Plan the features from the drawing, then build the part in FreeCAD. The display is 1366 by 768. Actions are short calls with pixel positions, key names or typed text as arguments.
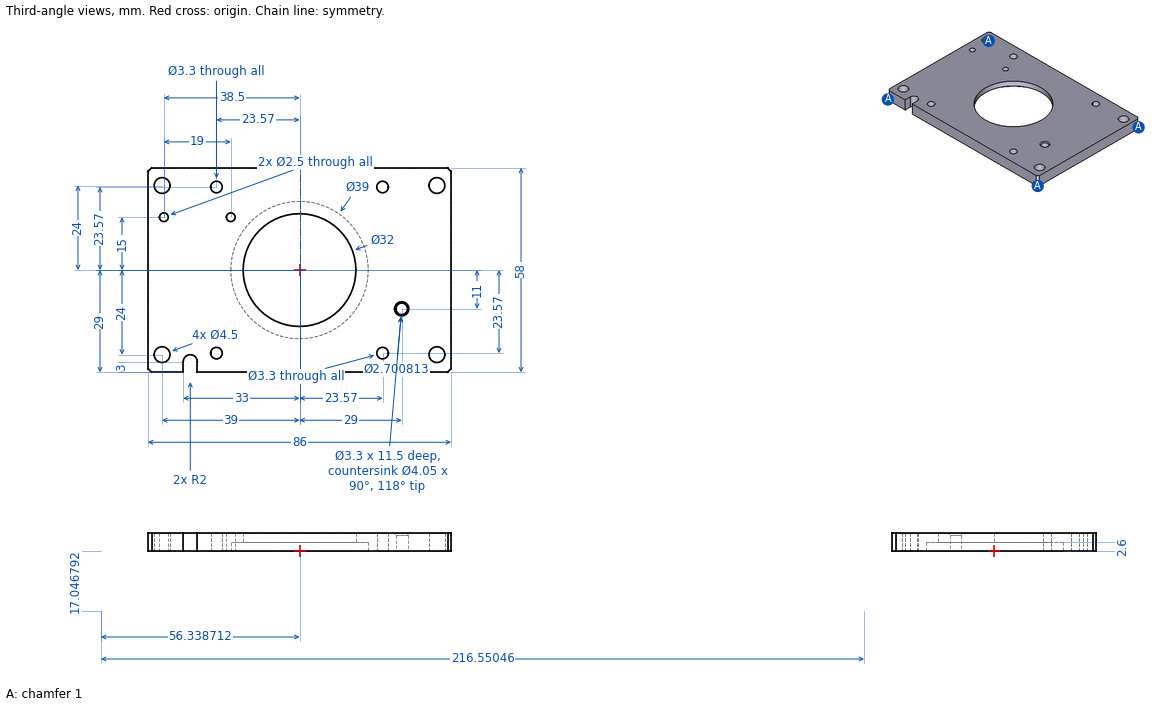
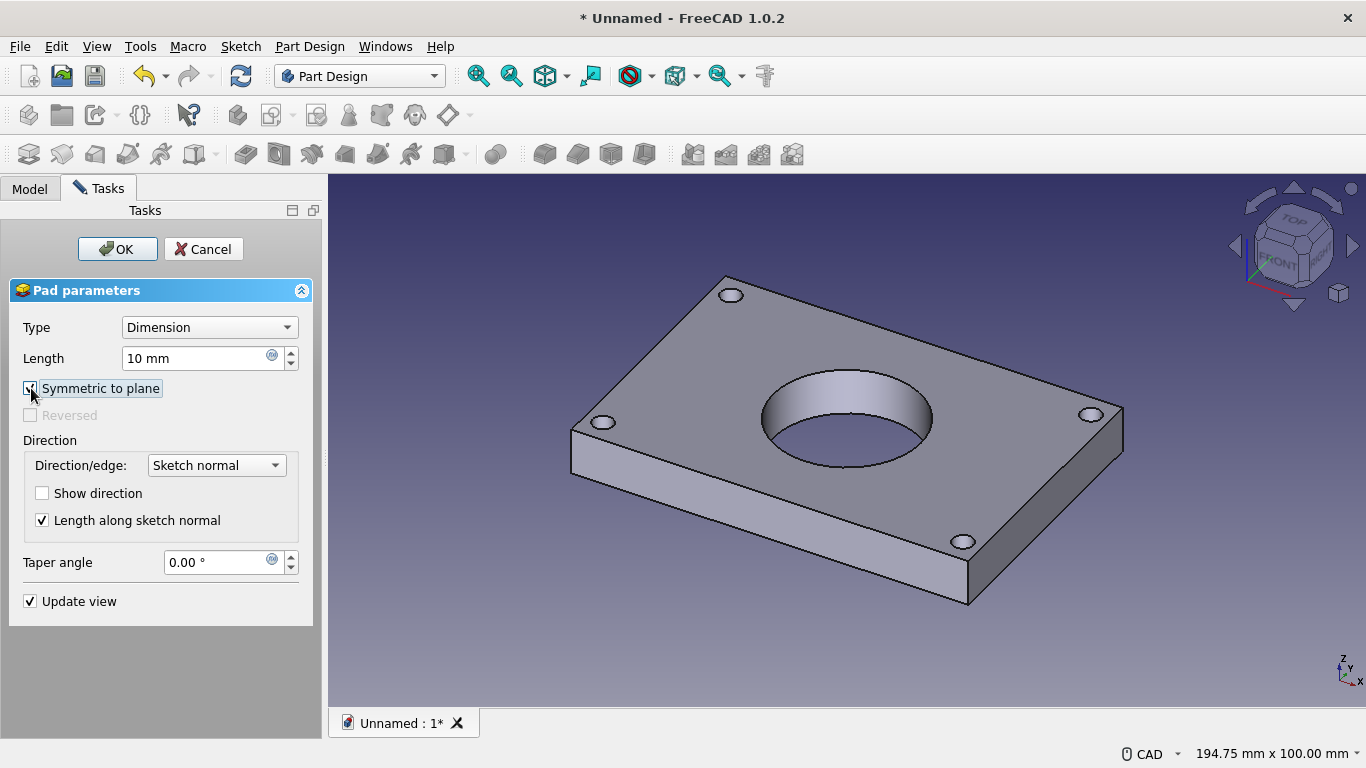
click(118, 249)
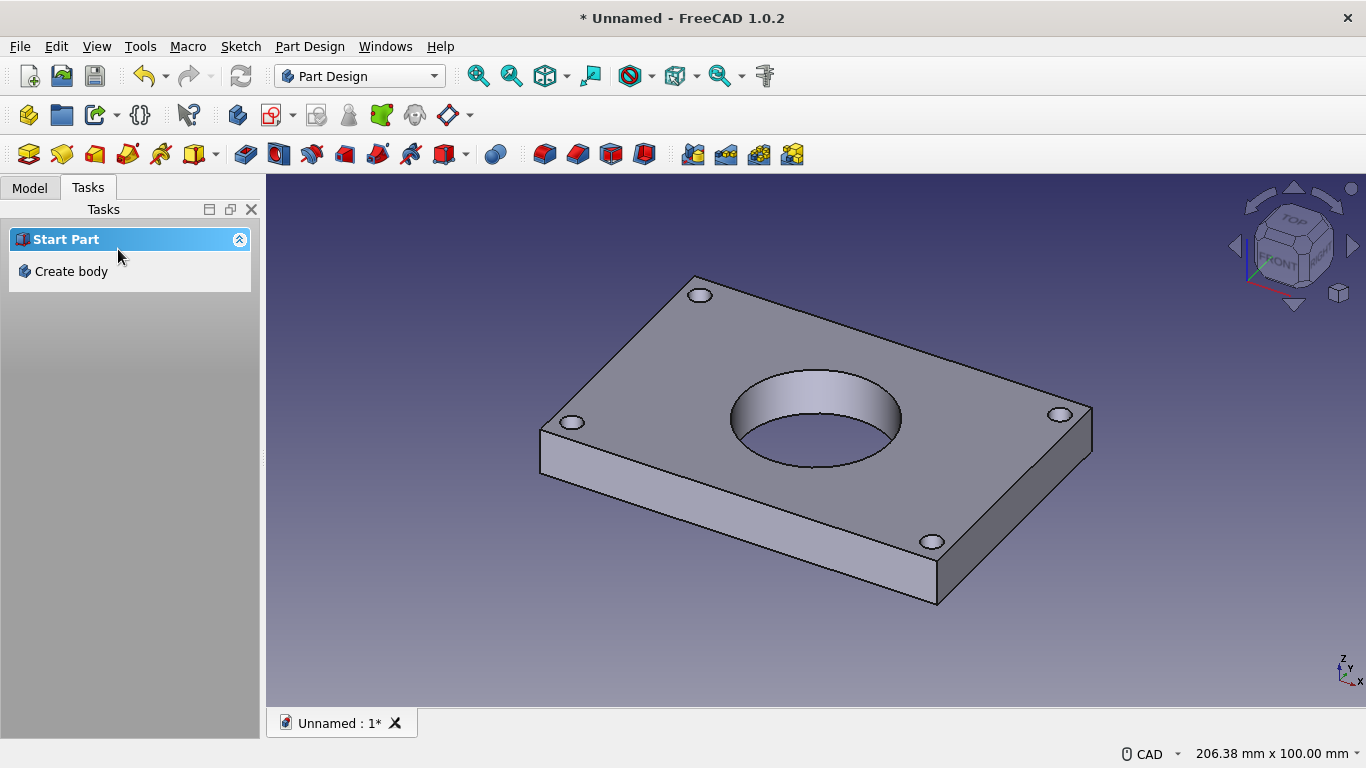
click(974, 411)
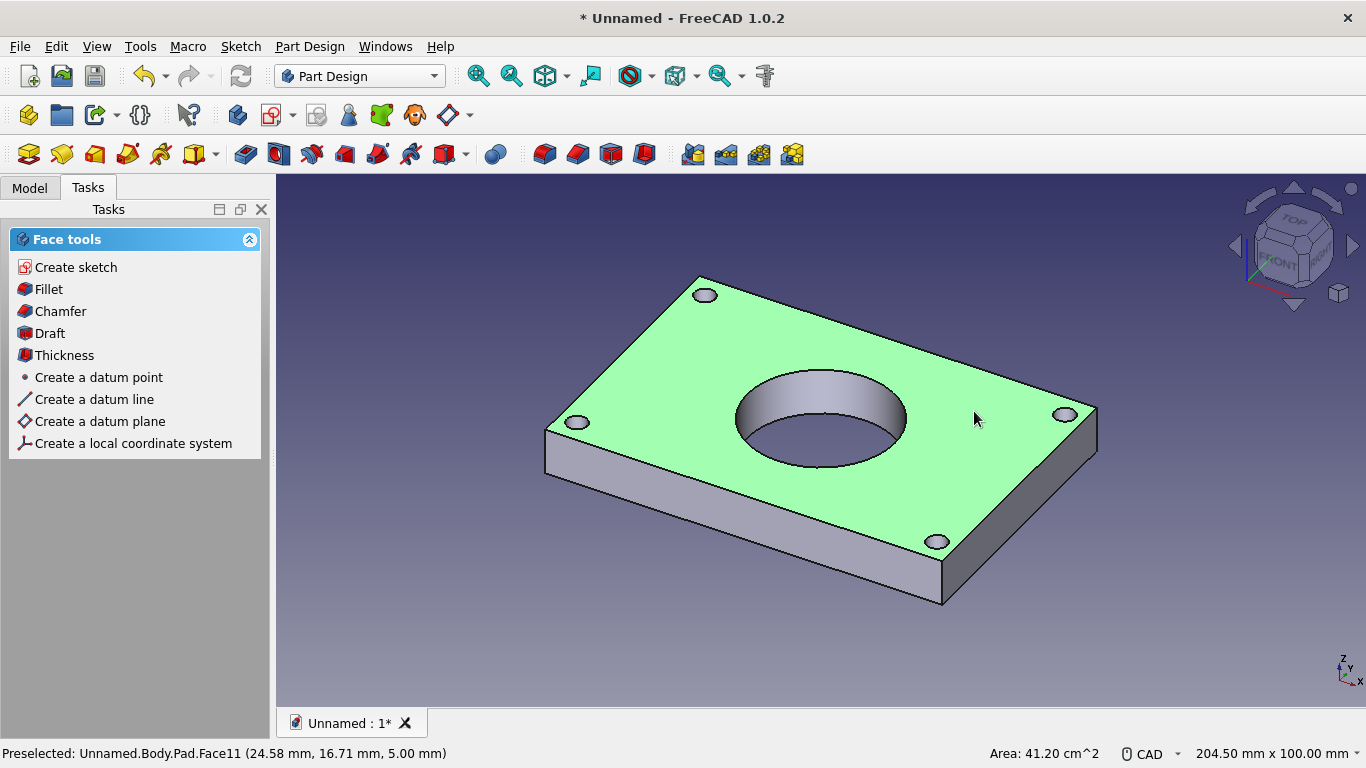
click(270, 116)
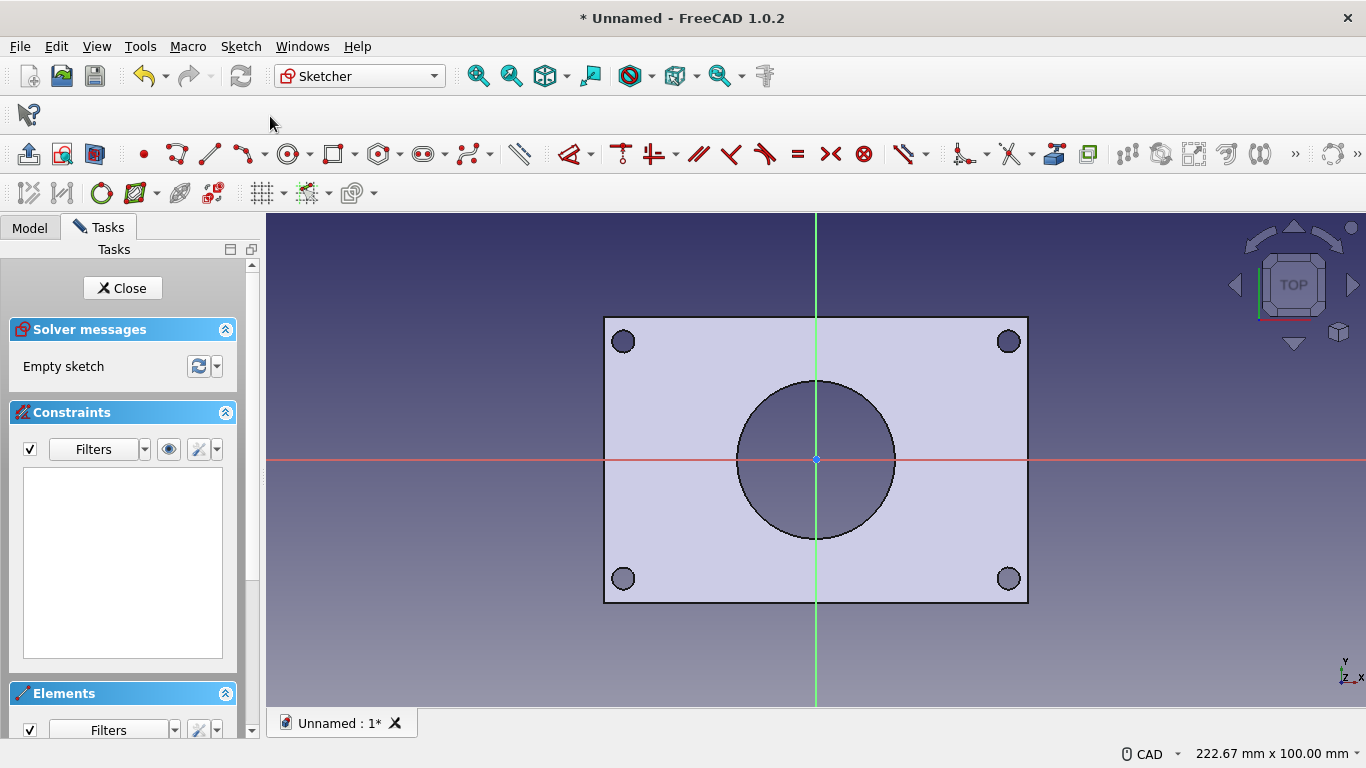
scroll(705, 403, up, 6)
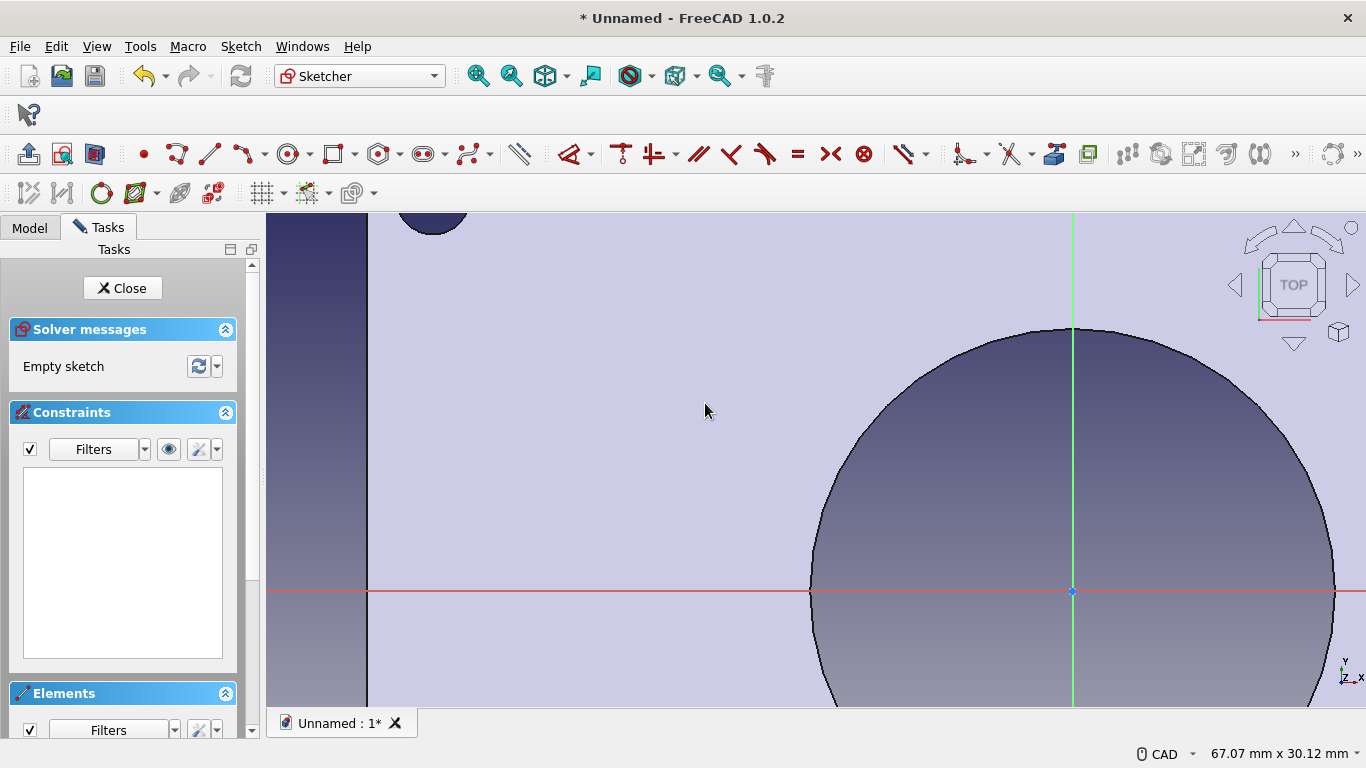
key(g)
key(c)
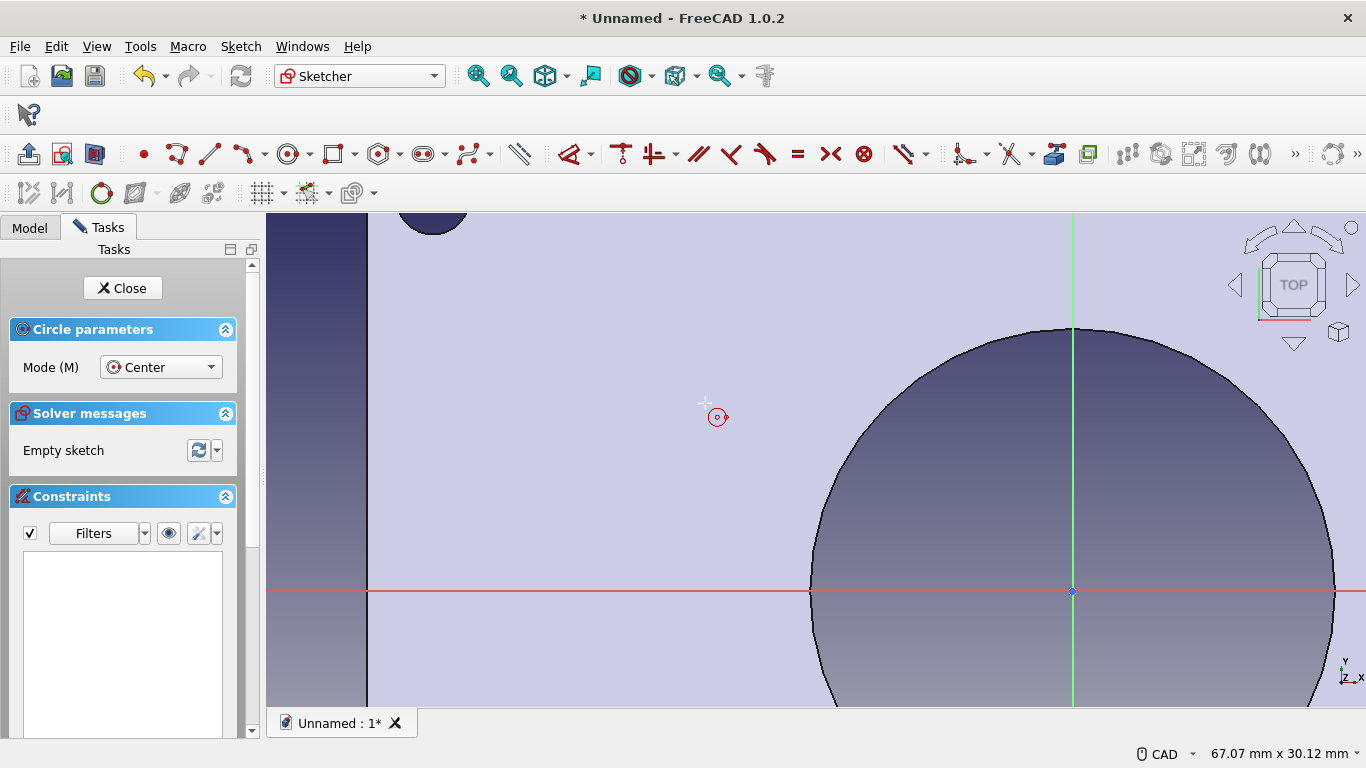
click(441, 345)
move(456, 331)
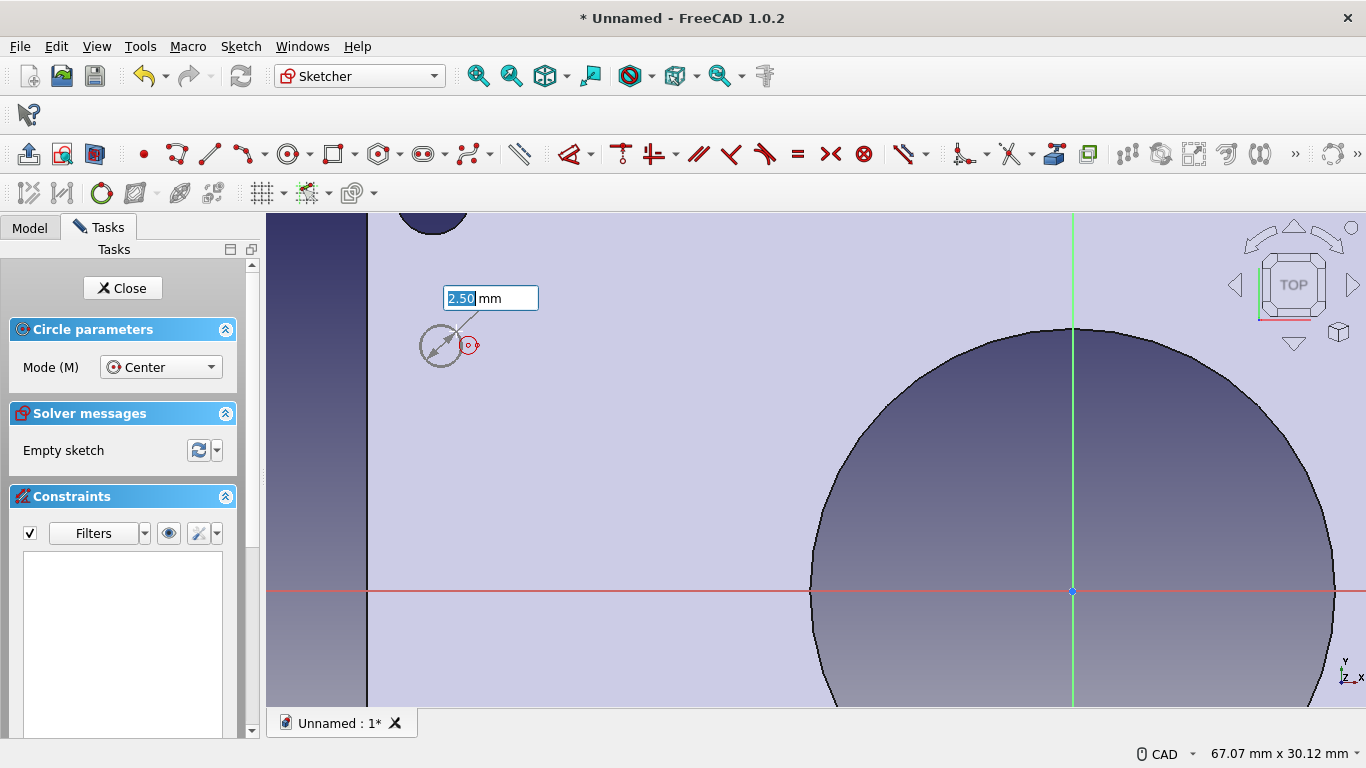
text(2.5)
key(Return)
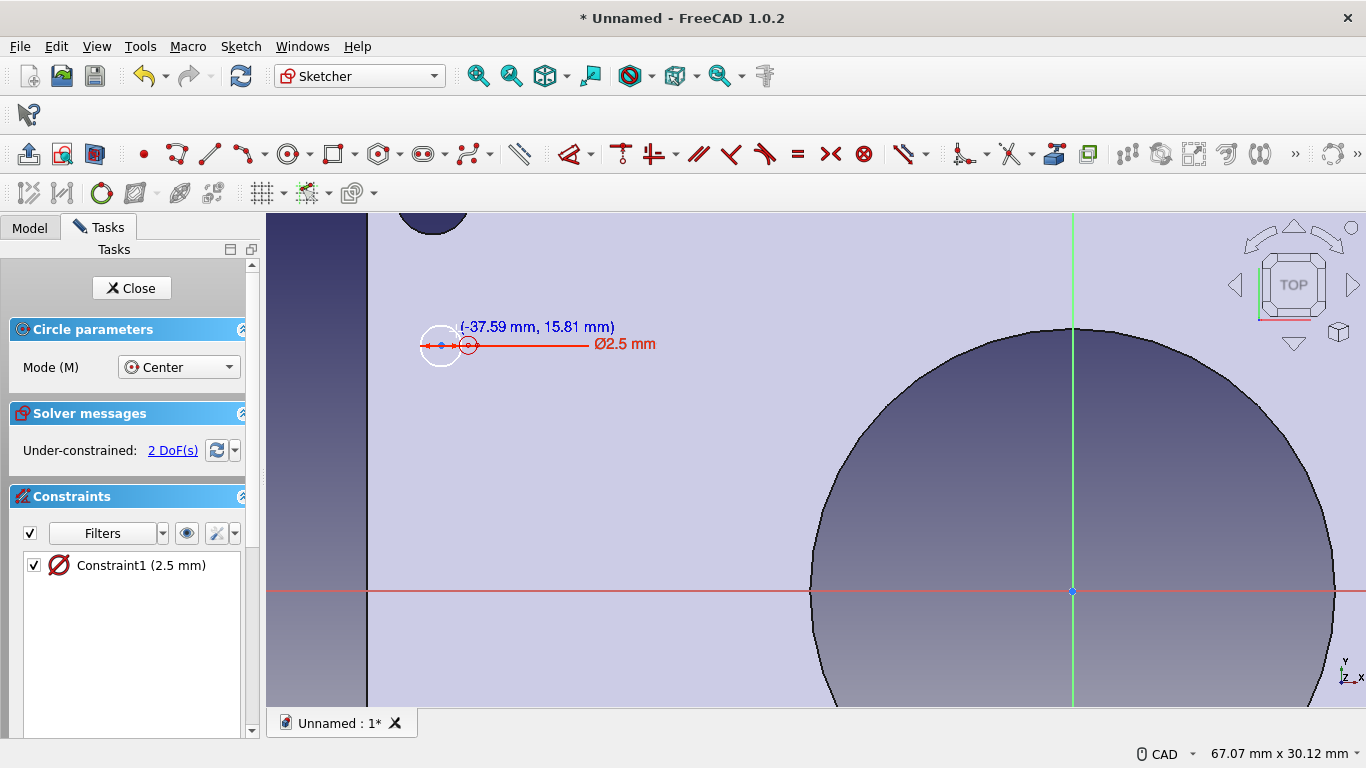
click(753, 345)
move(767, 331)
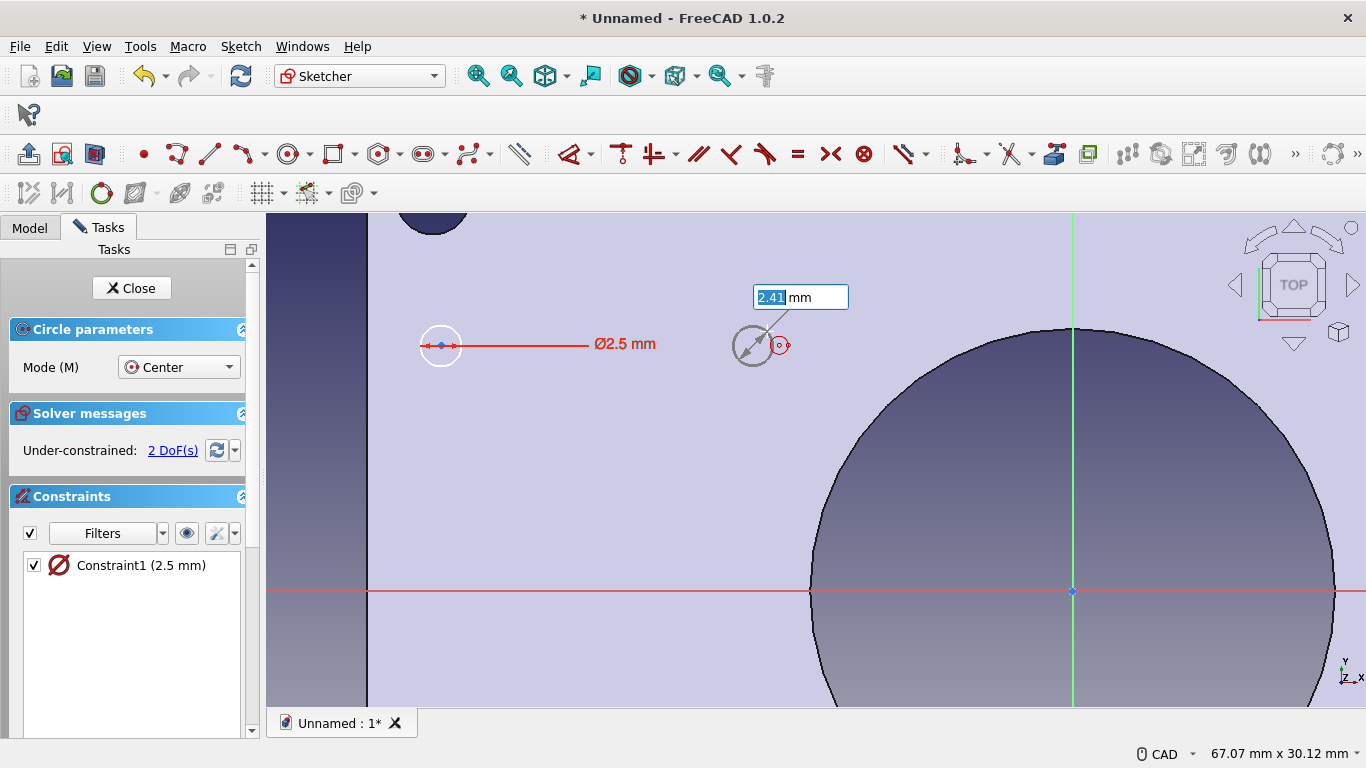
text(2.5)
key(Return)
key(Escape)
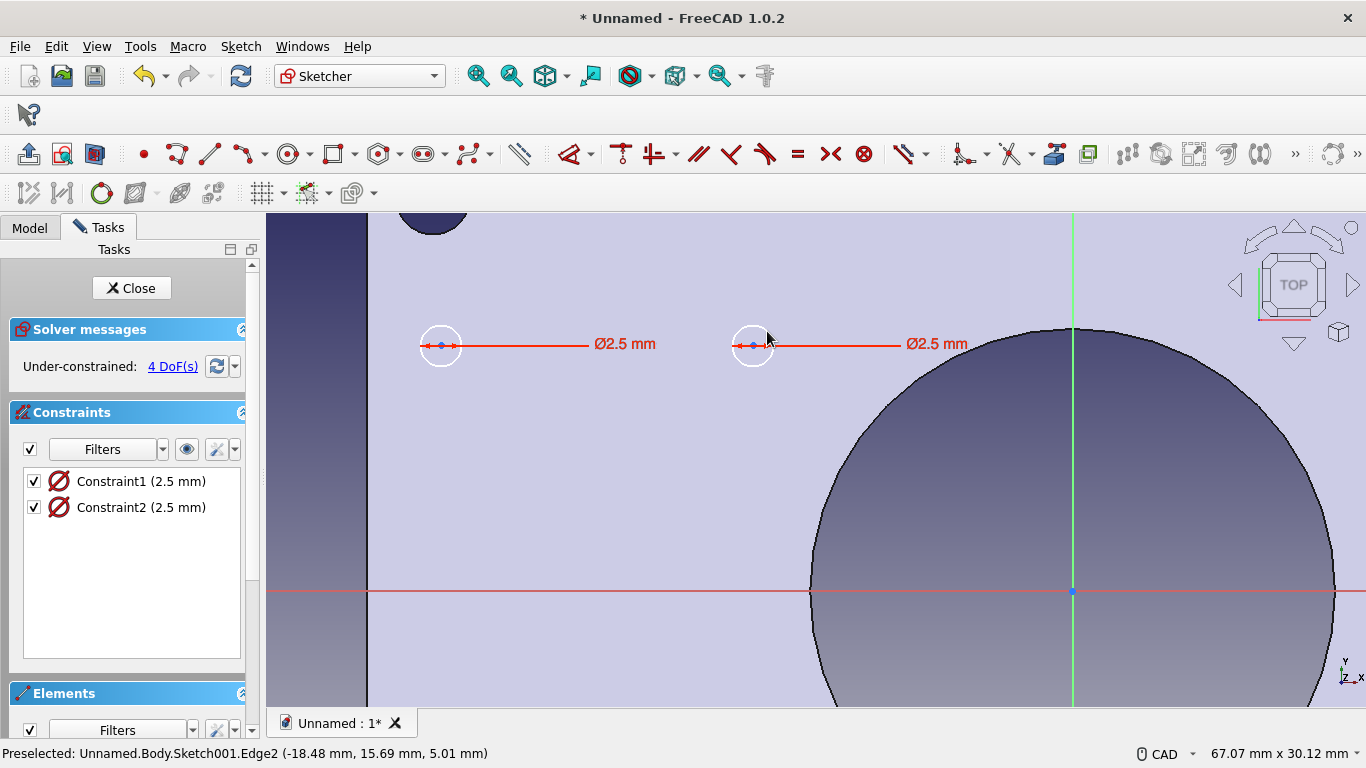
click(441, 346)